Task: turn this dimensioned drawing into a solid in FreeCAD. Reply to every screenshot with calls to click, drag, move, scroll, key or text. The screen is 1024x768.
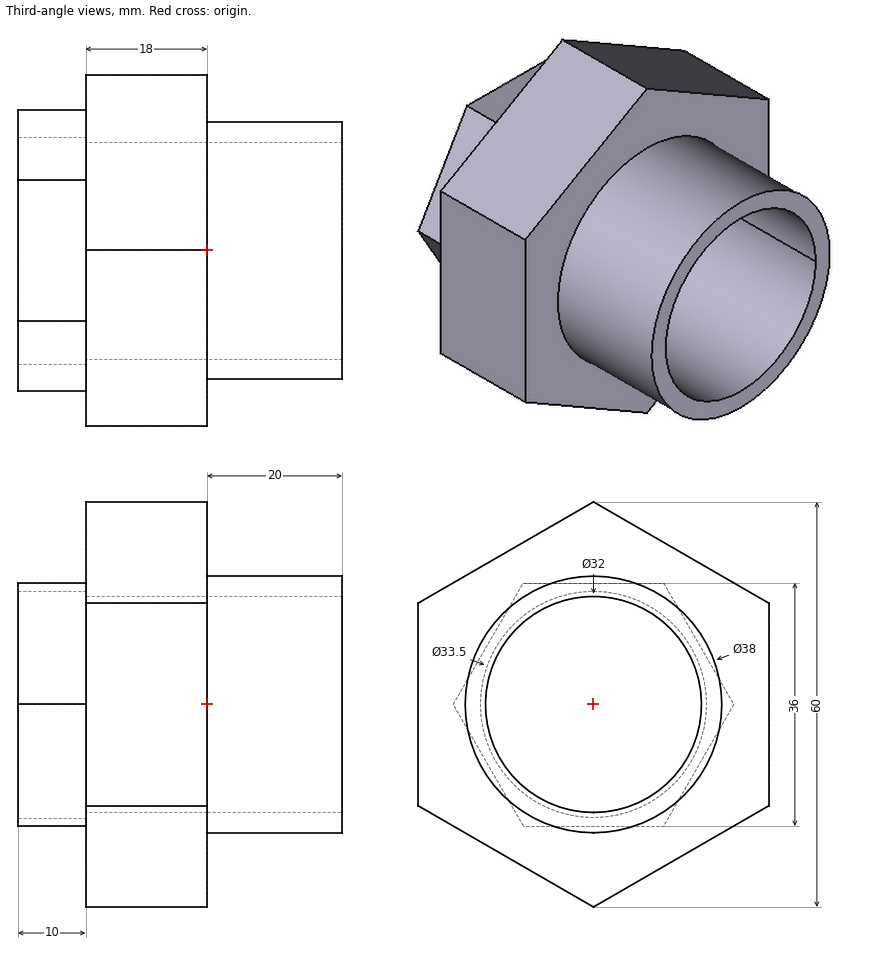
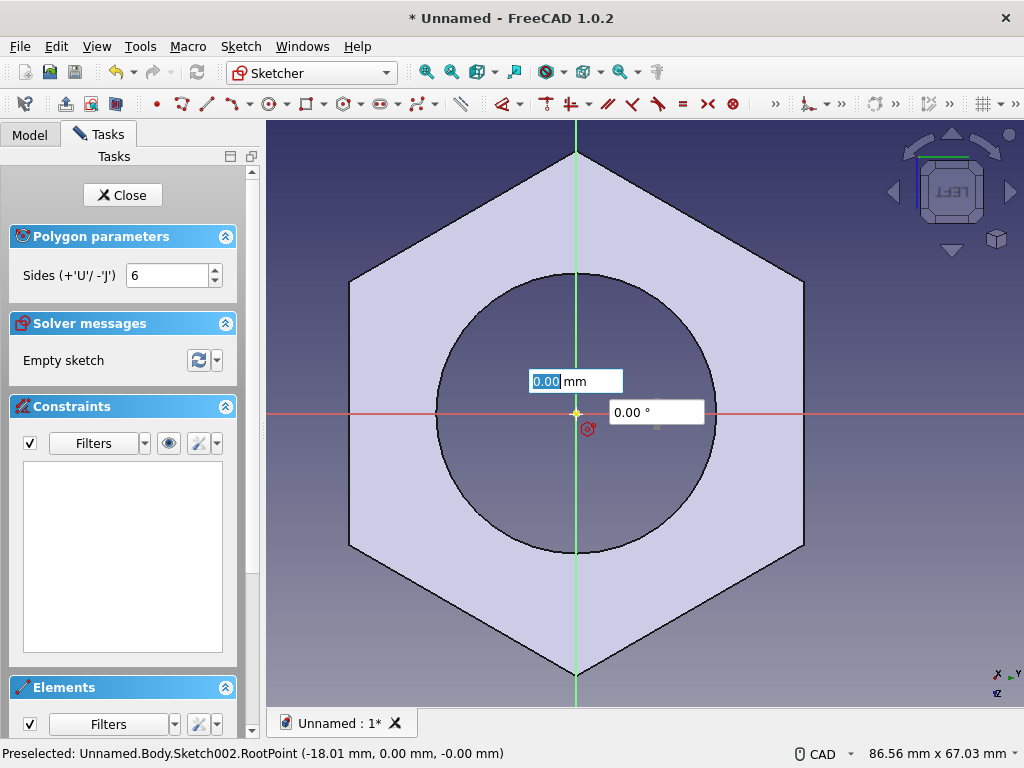
click(758, 414)
right_click(758, 414)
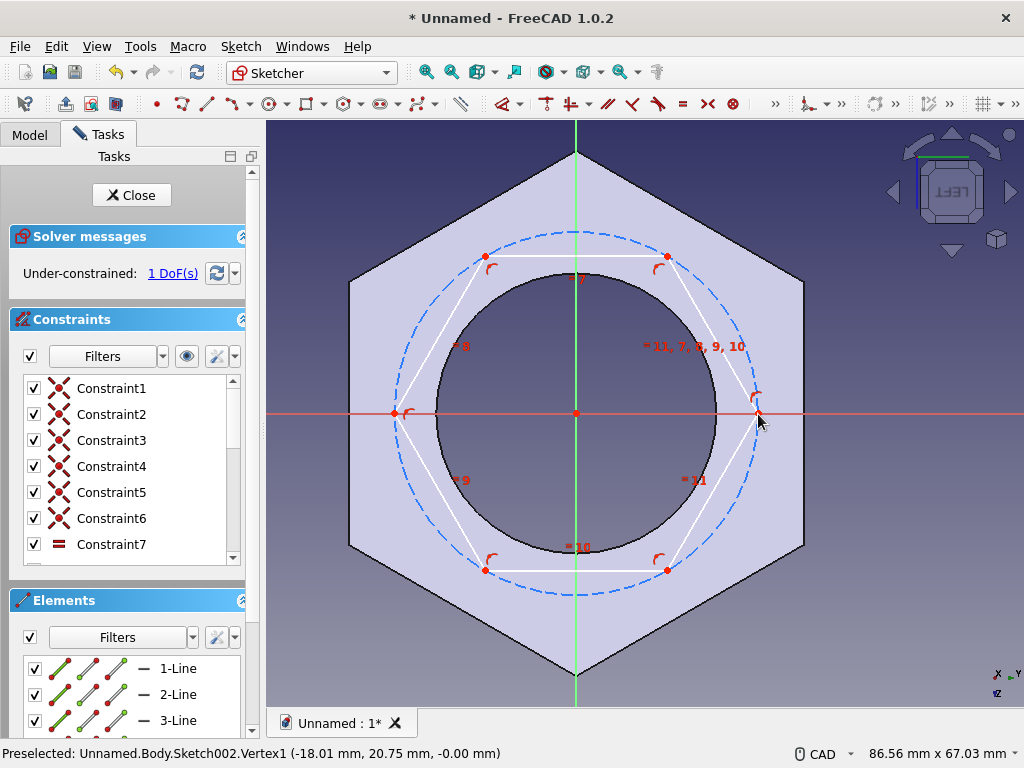
key(g)
key(c)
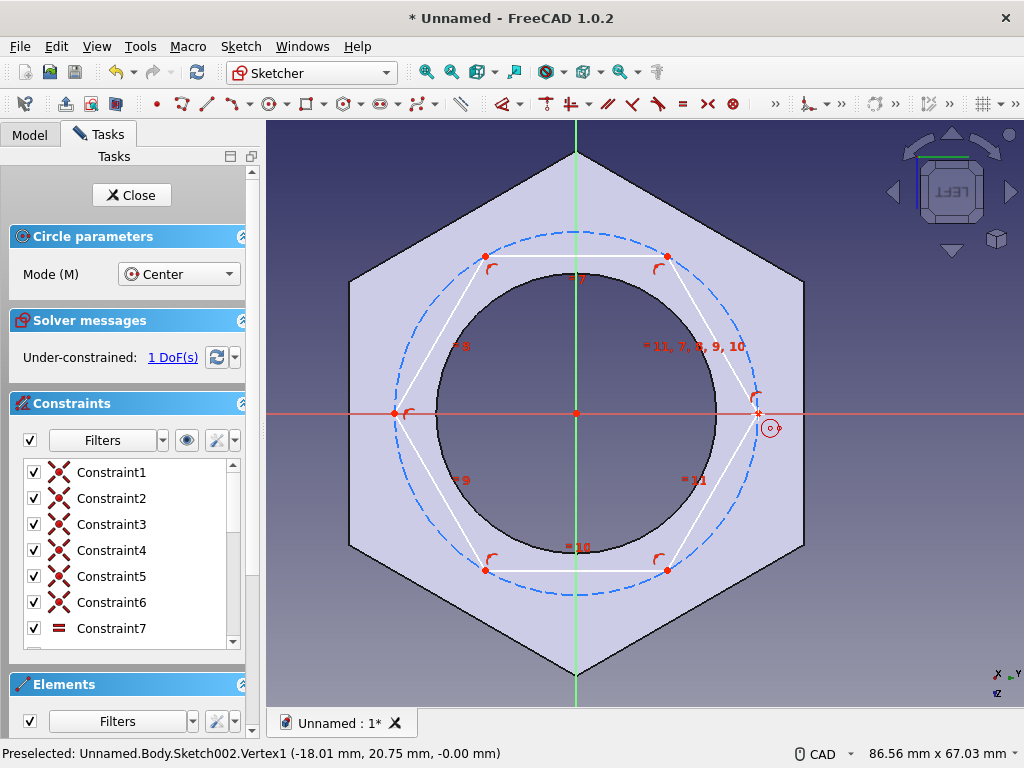
click(576, 414)
click(680, 310)
key(Escape)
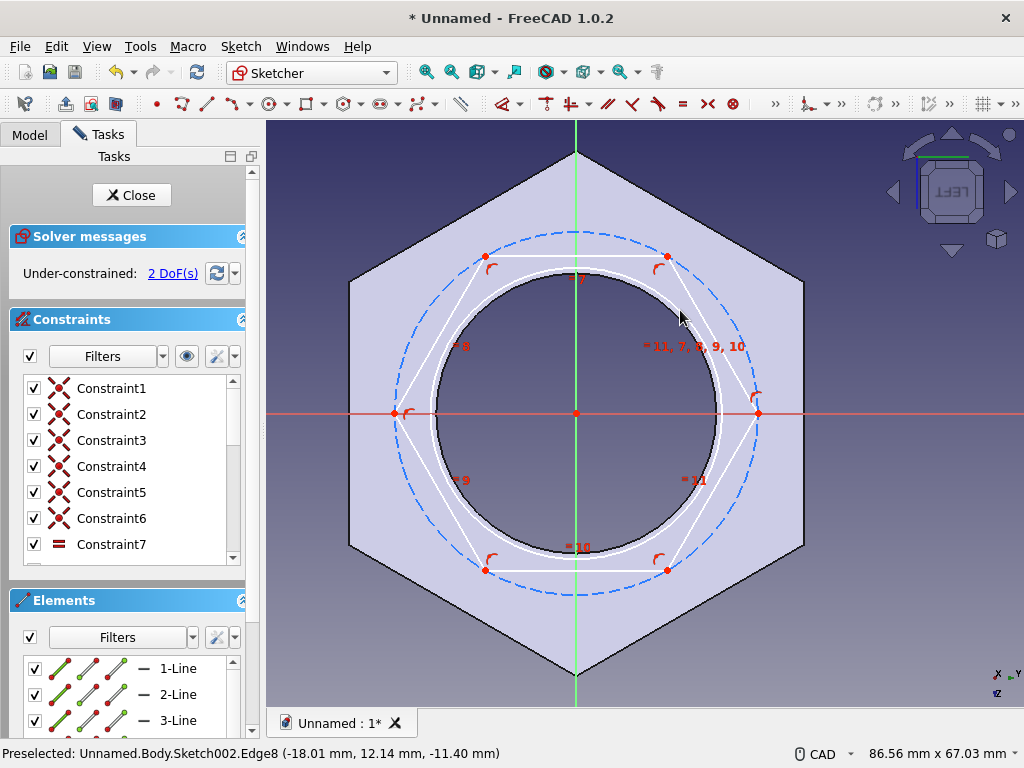
click(679, 310)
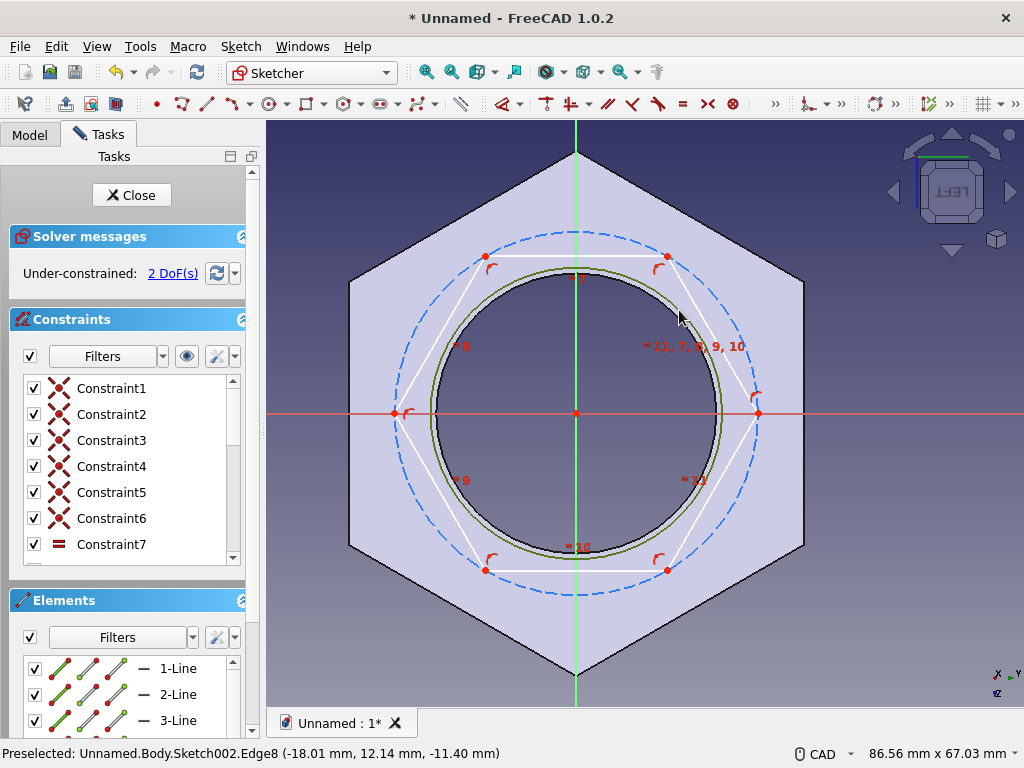
key(k)
key(o)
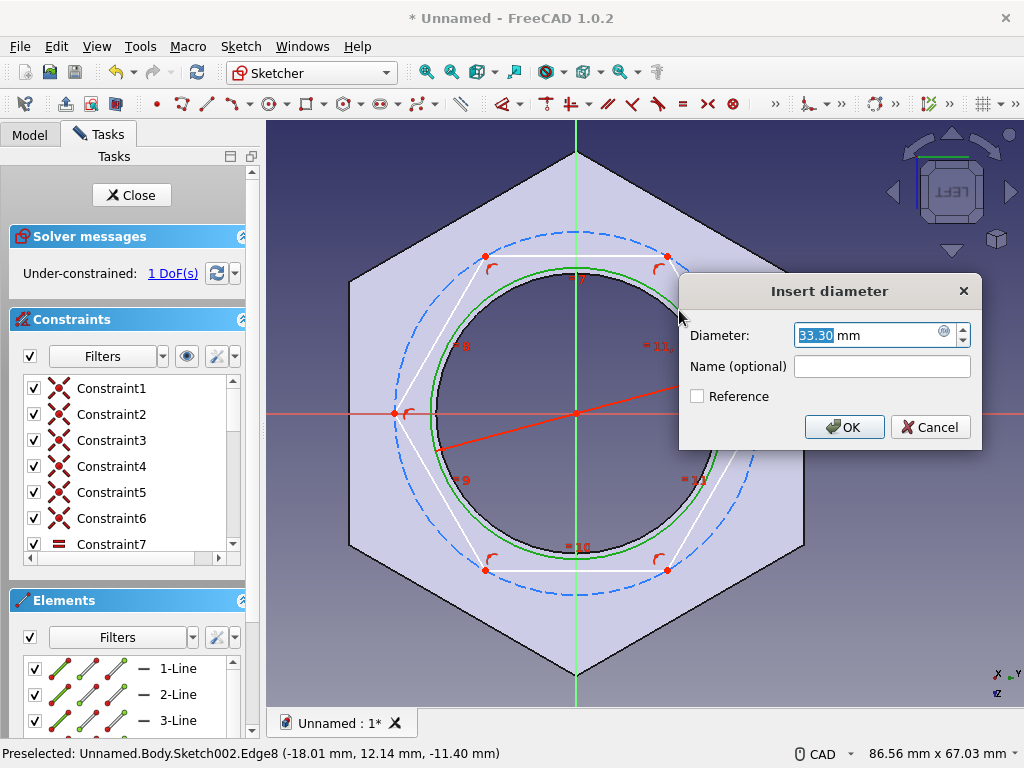
text(33.5)
key(Return)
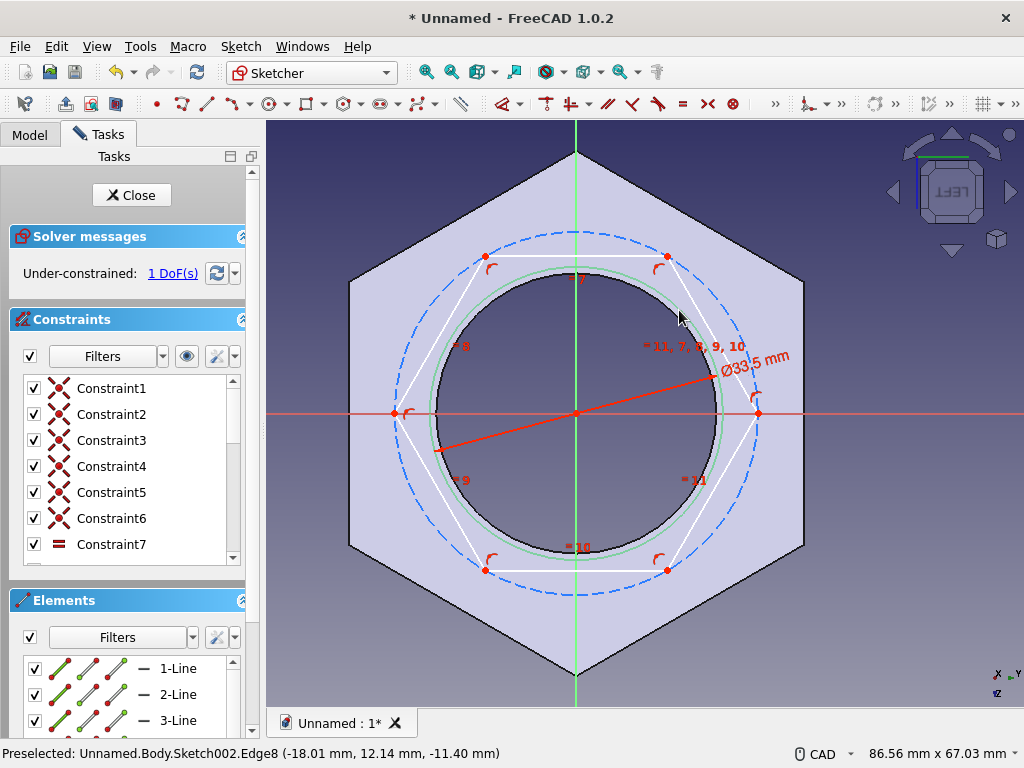
click(485, 571)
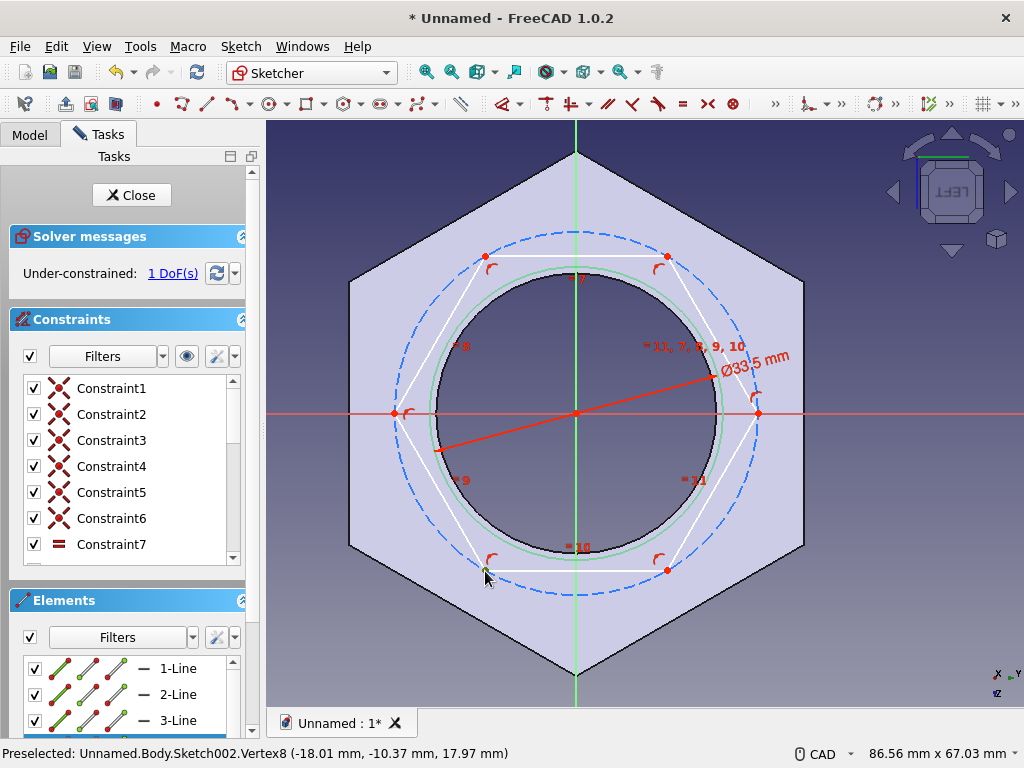
click(667, 256)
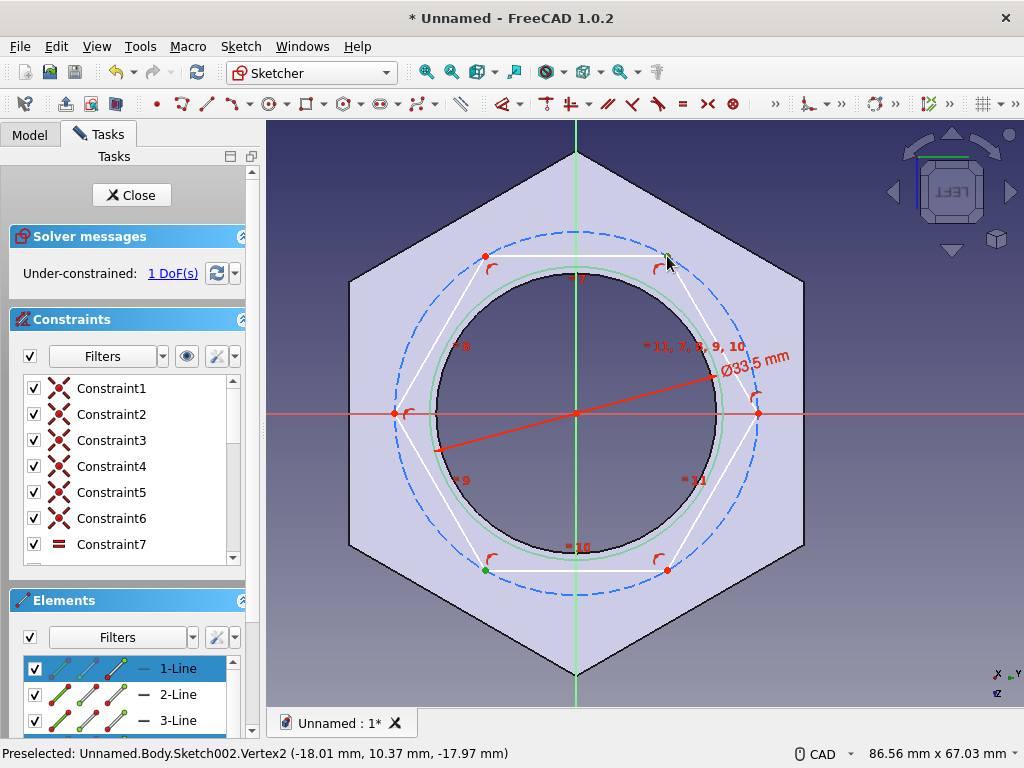
click(520, 104)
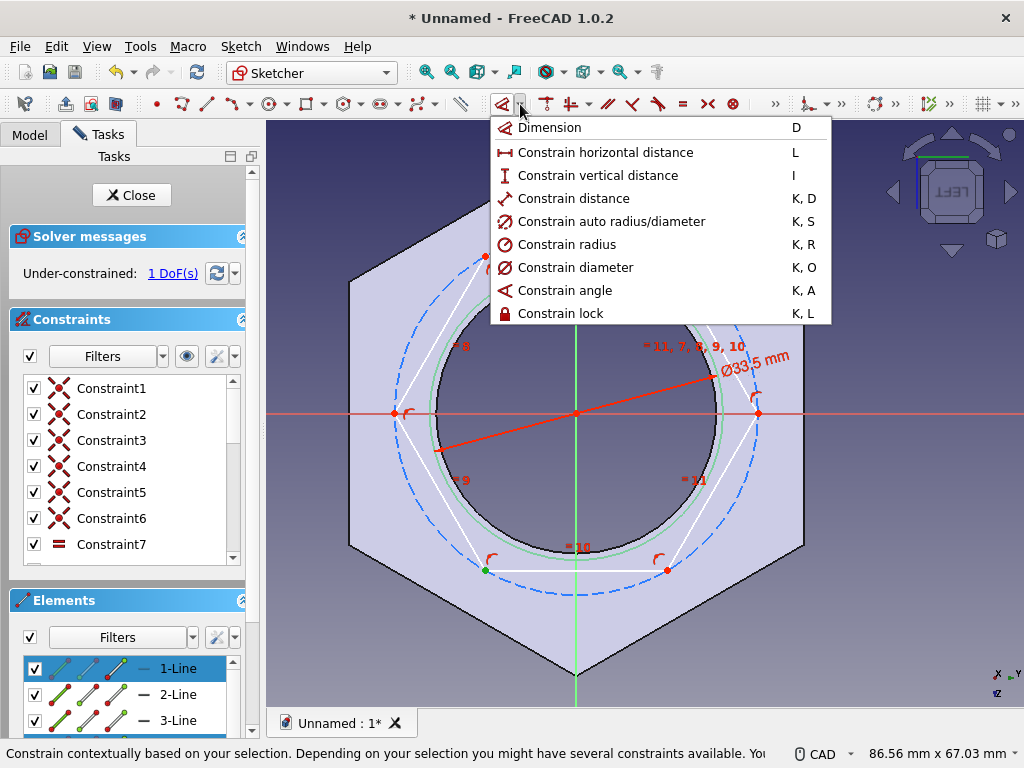
click(661, 176)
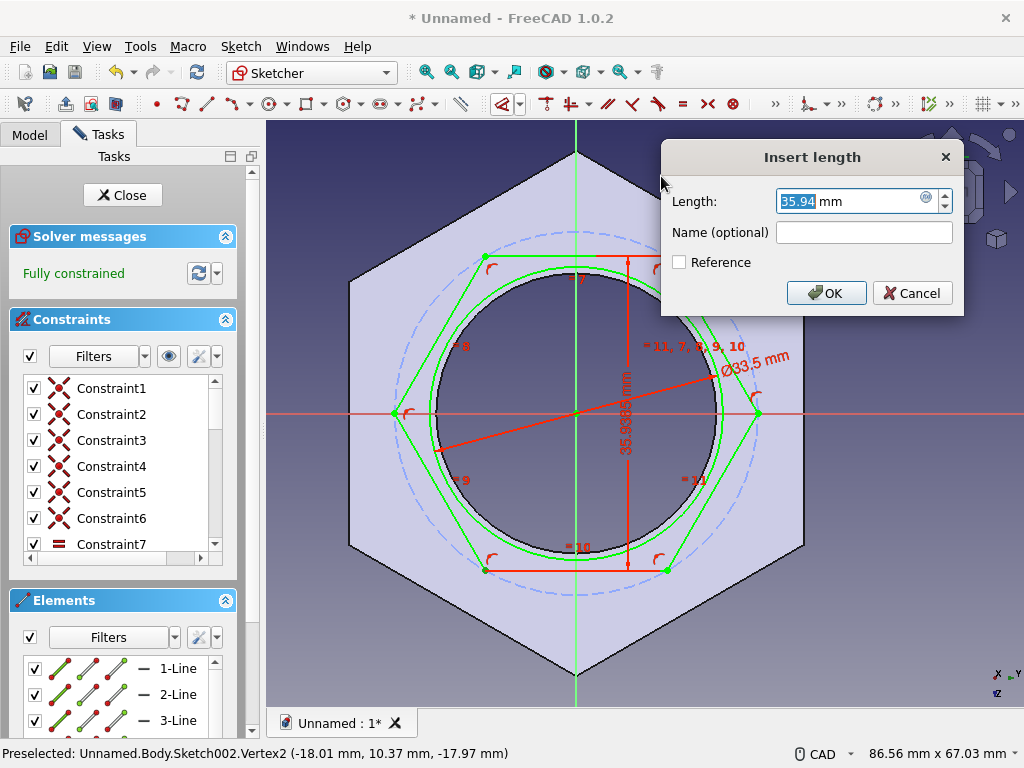
text(36)
key(Return)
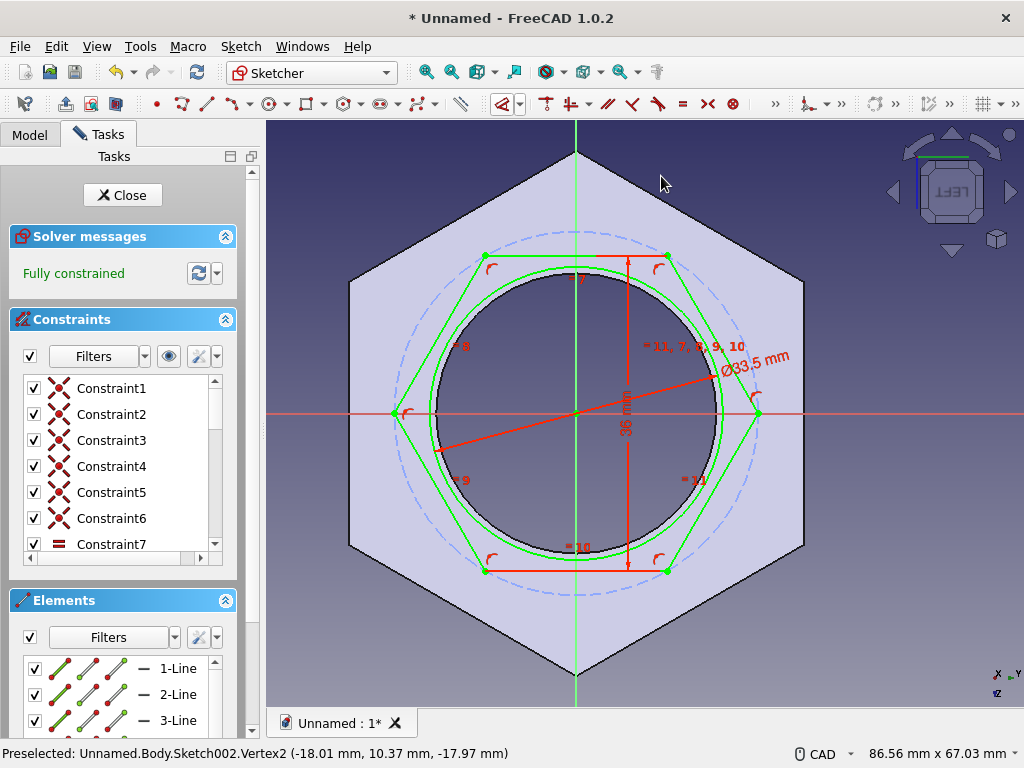
click(123, 195)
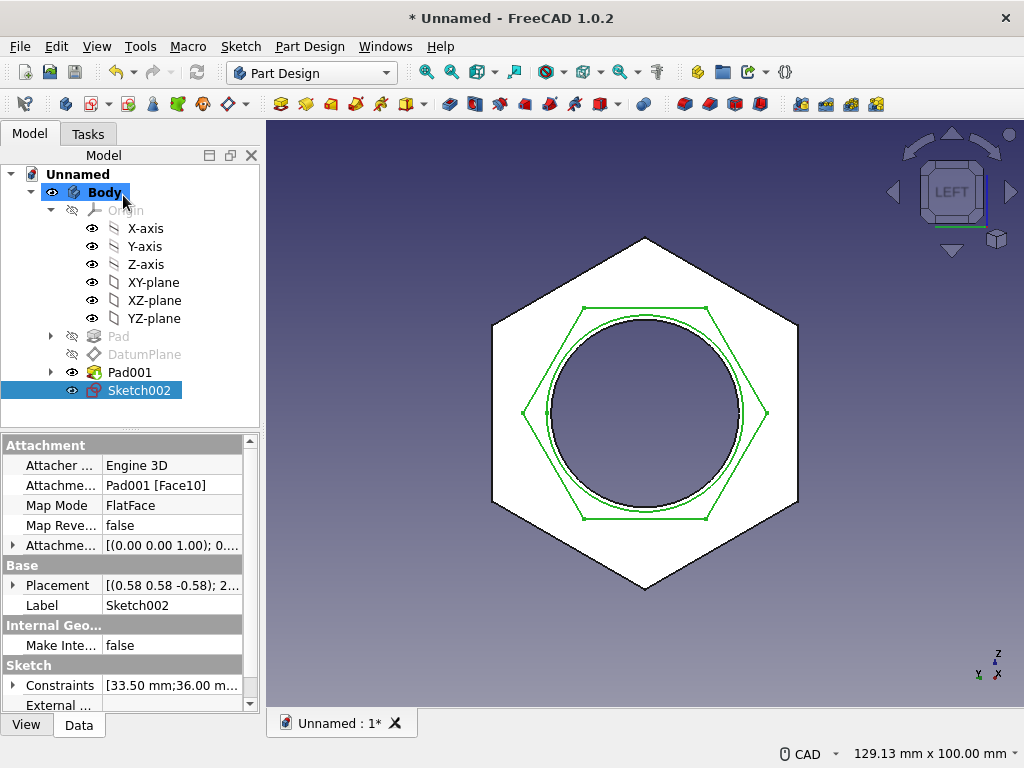
click(281, 104)